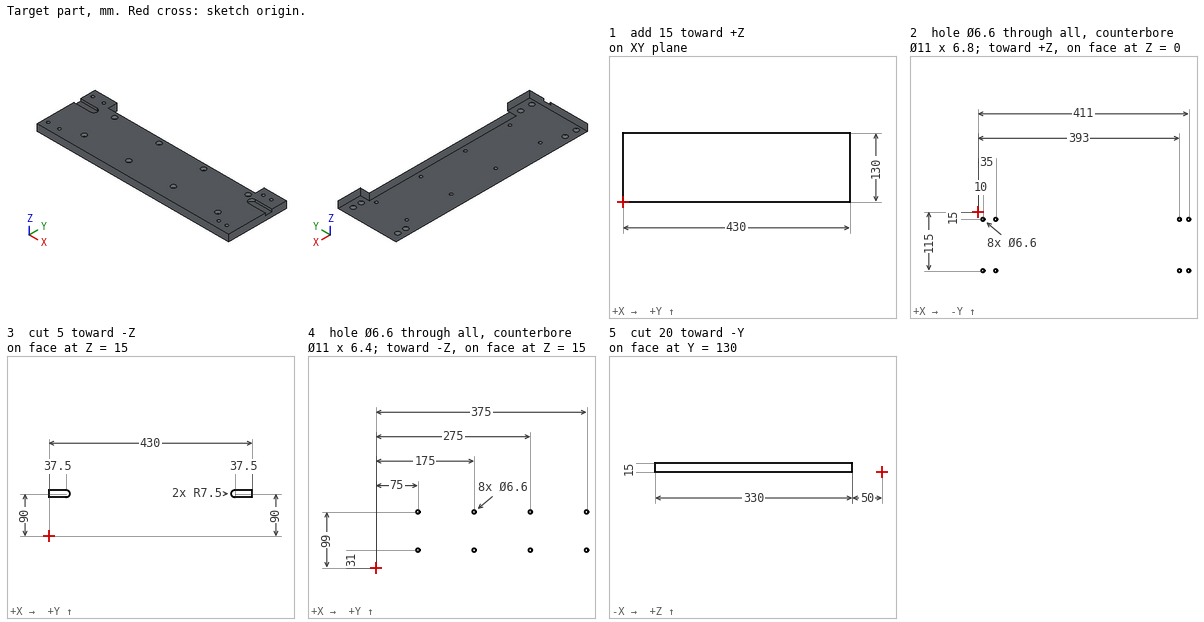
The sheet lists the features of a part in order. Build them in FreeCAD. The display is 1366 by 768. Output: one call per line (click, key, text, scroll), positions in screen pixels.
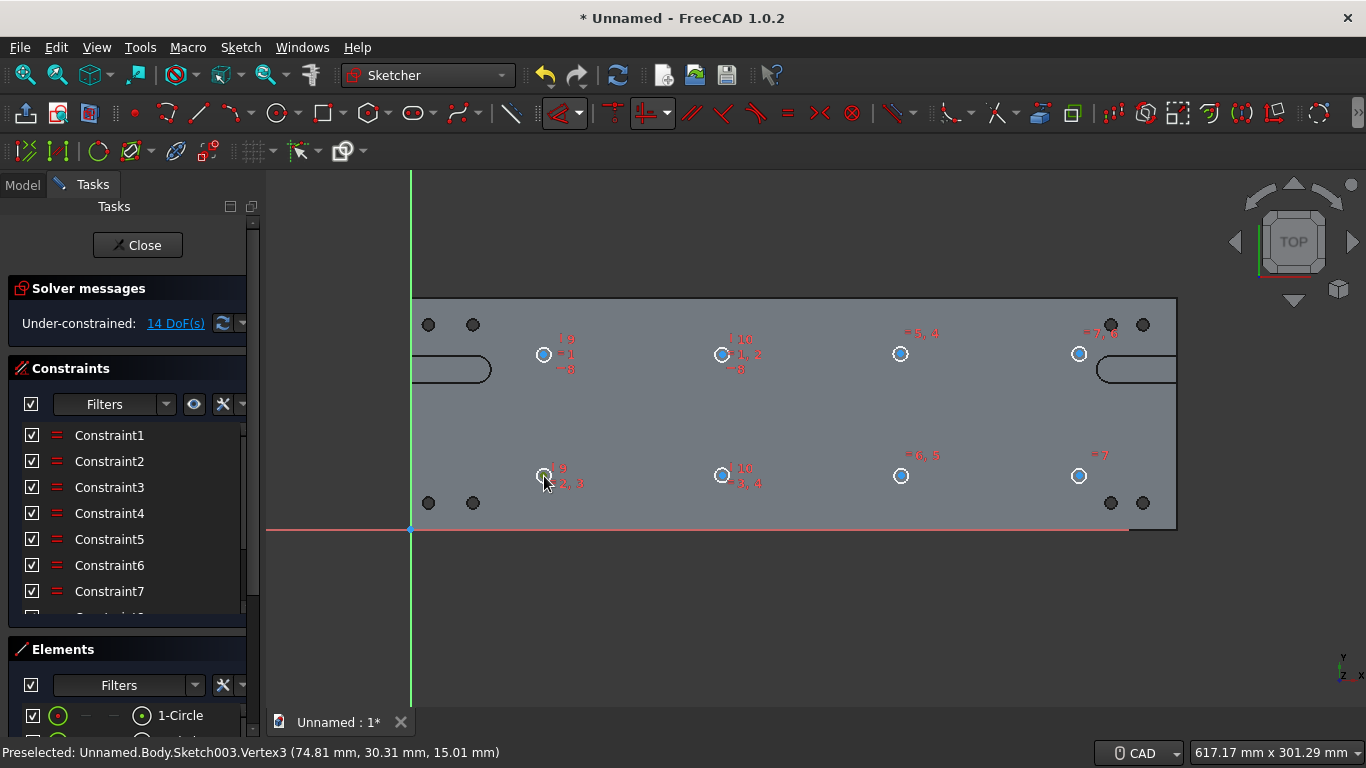
click(722, 475)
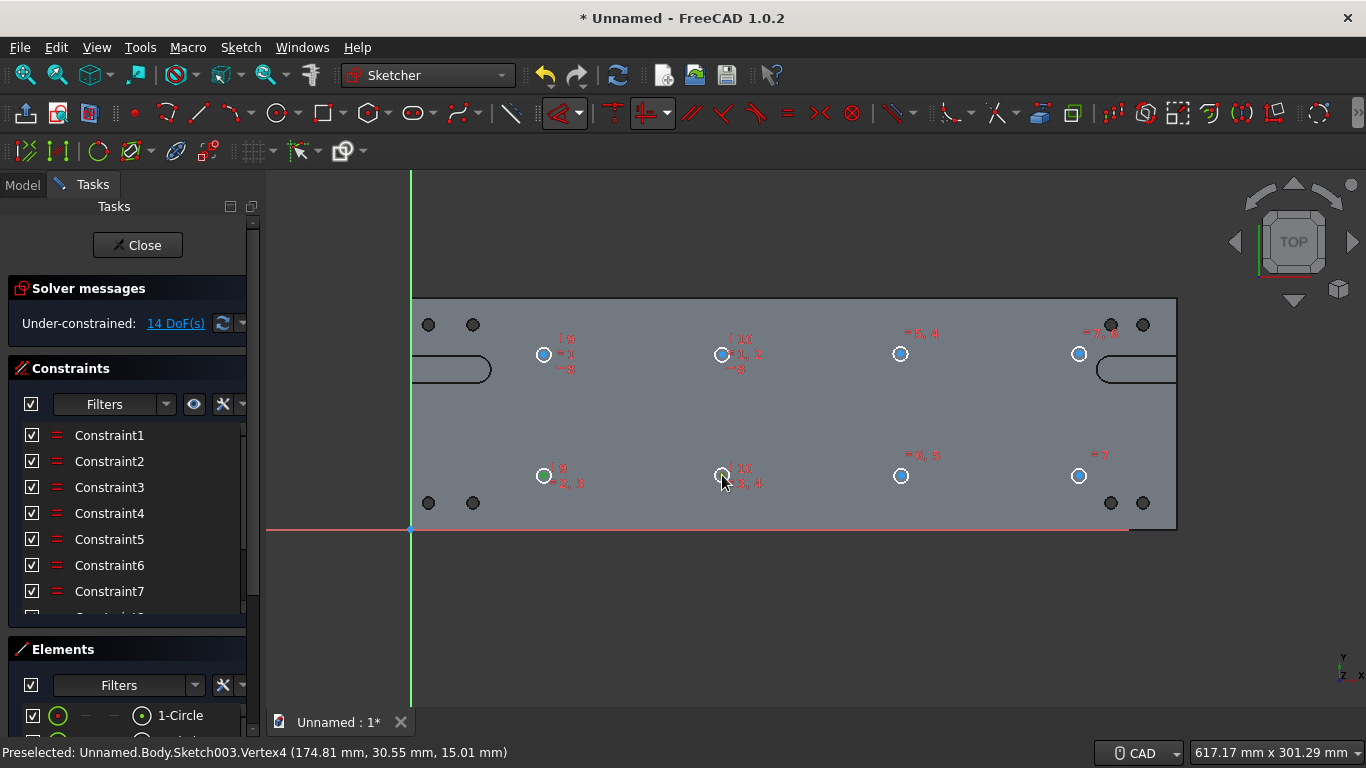
key(h)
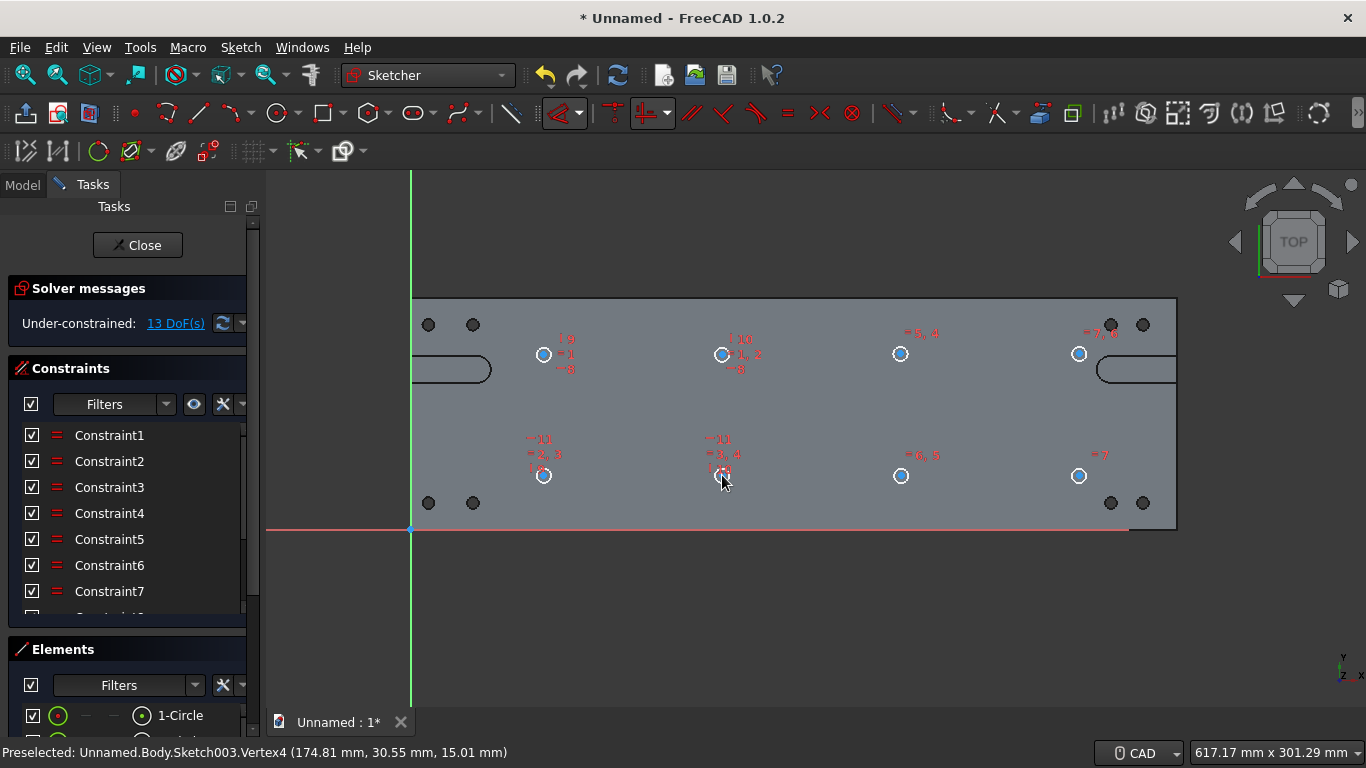
click(722, 355)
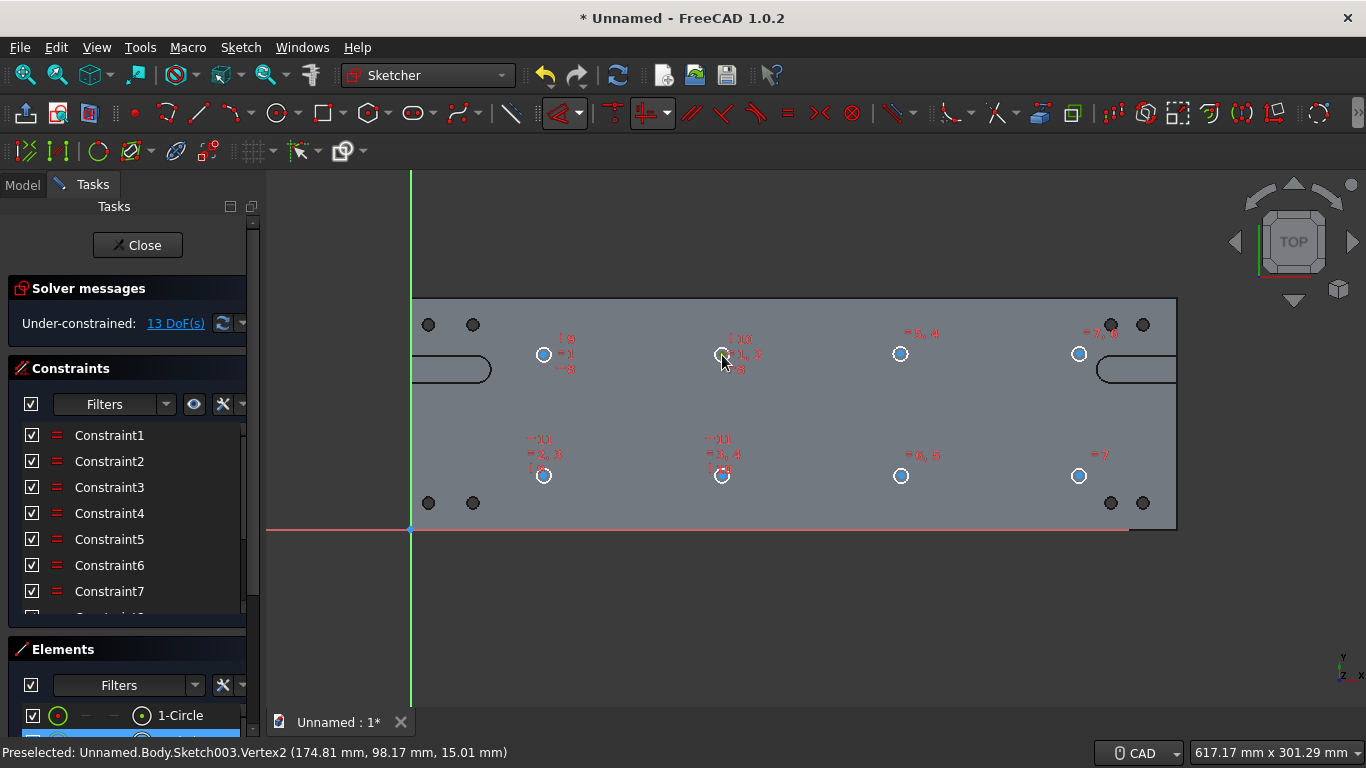
click(900, 354)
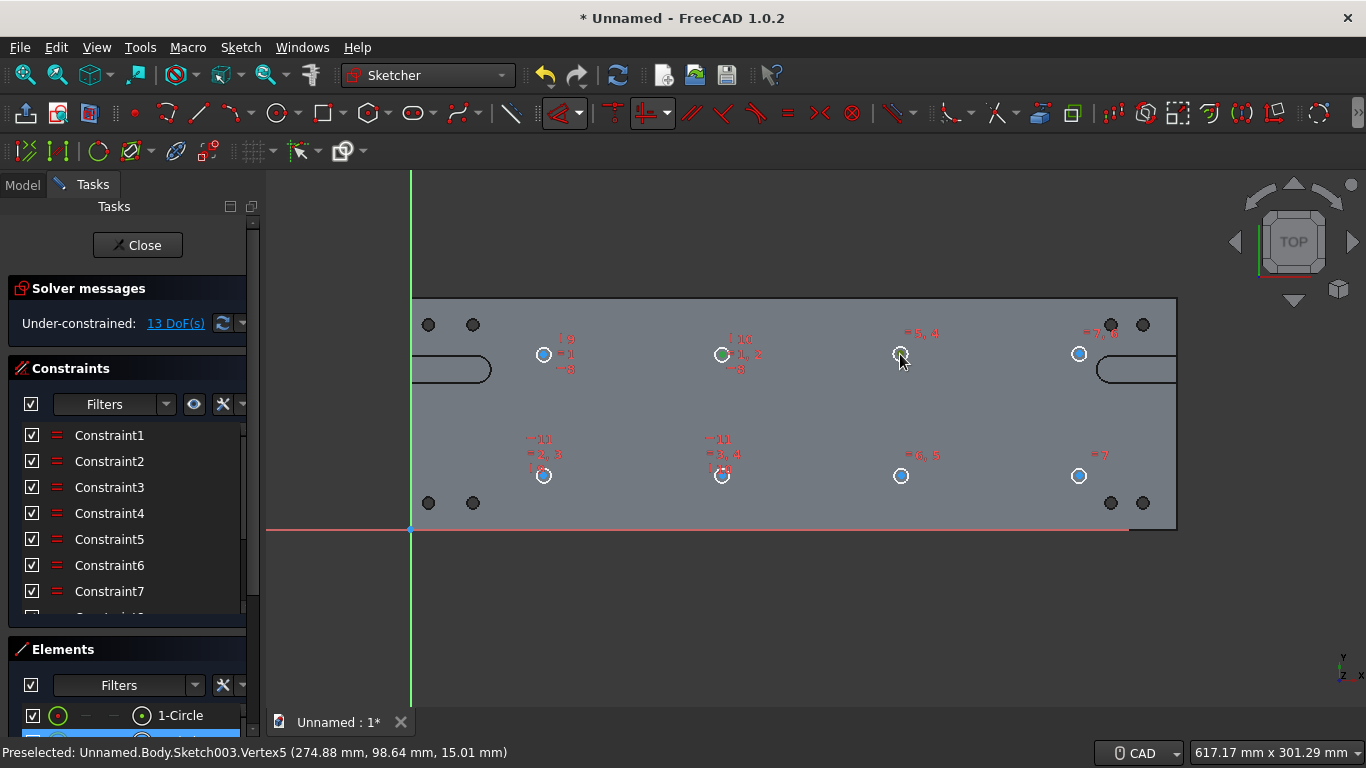
key(h)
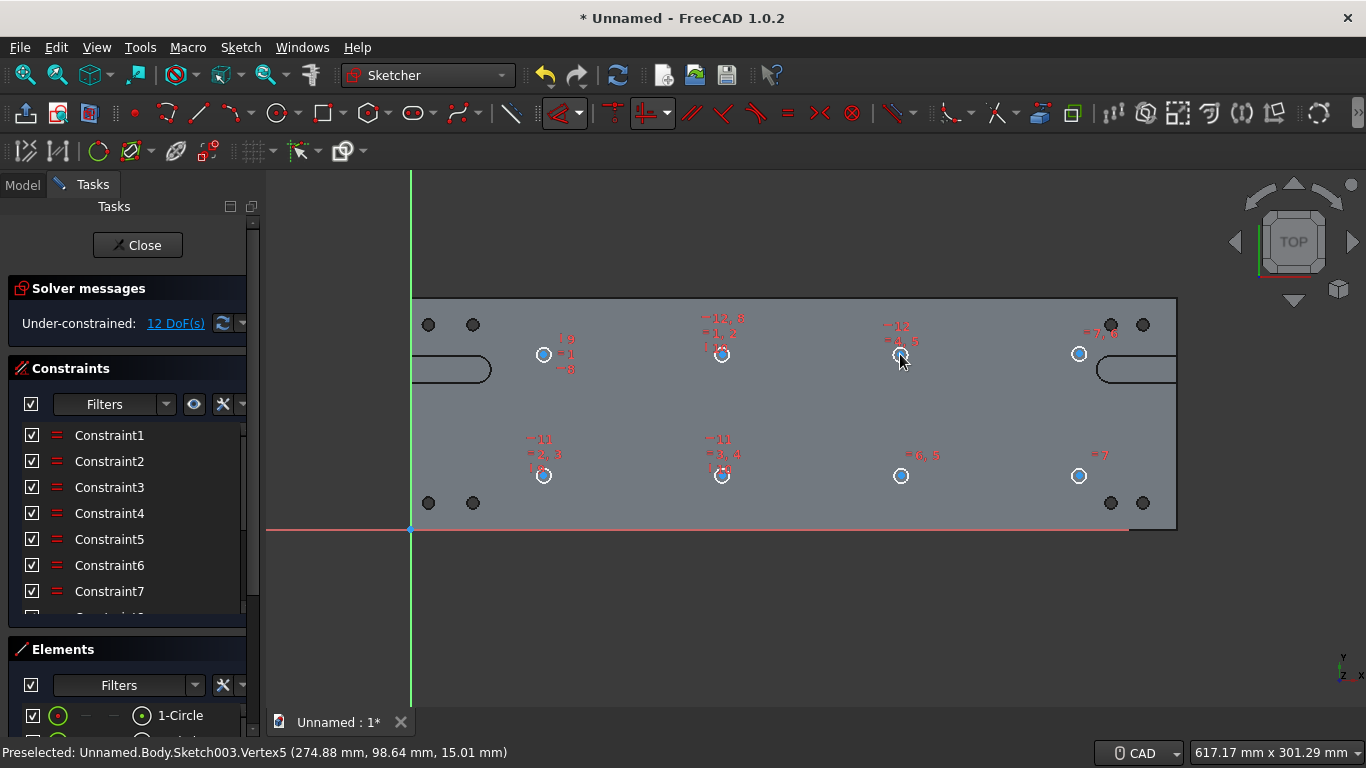
click(900, 355)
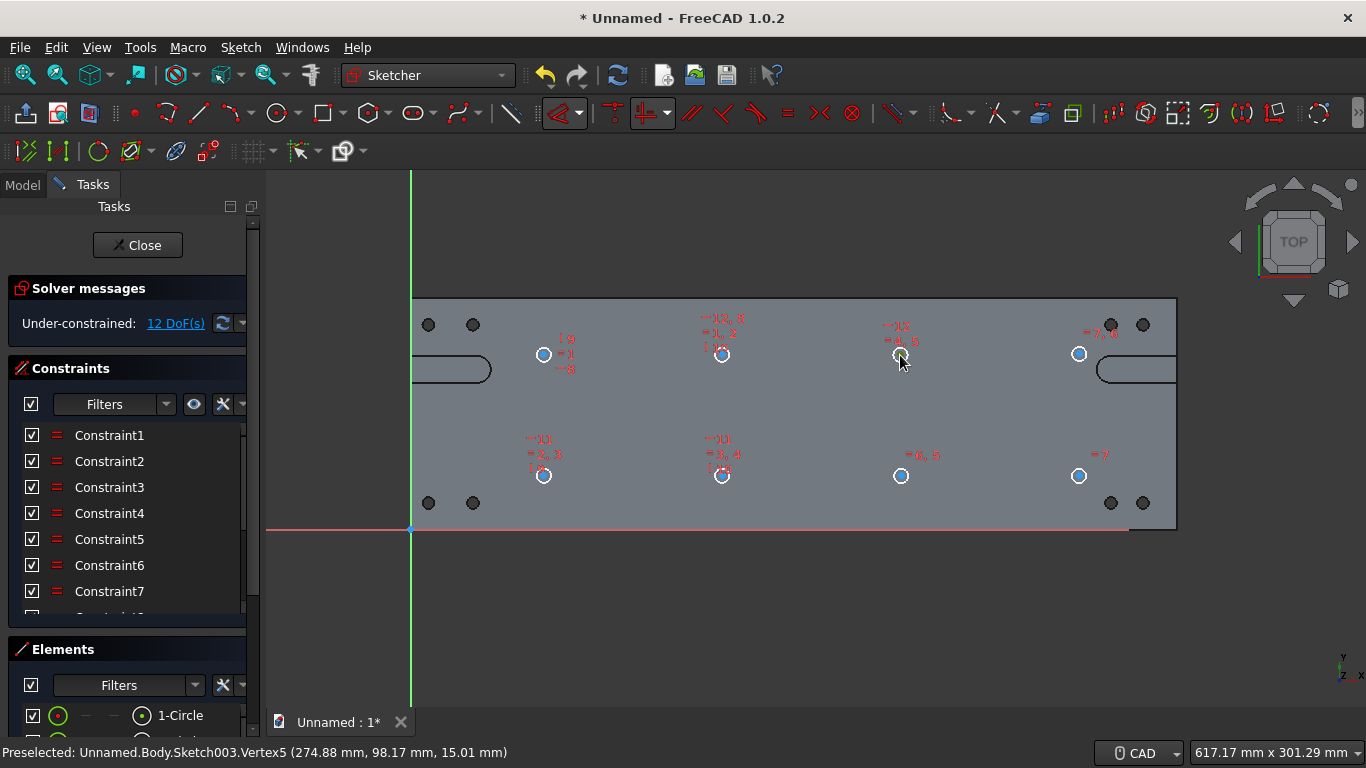
click(901, 476)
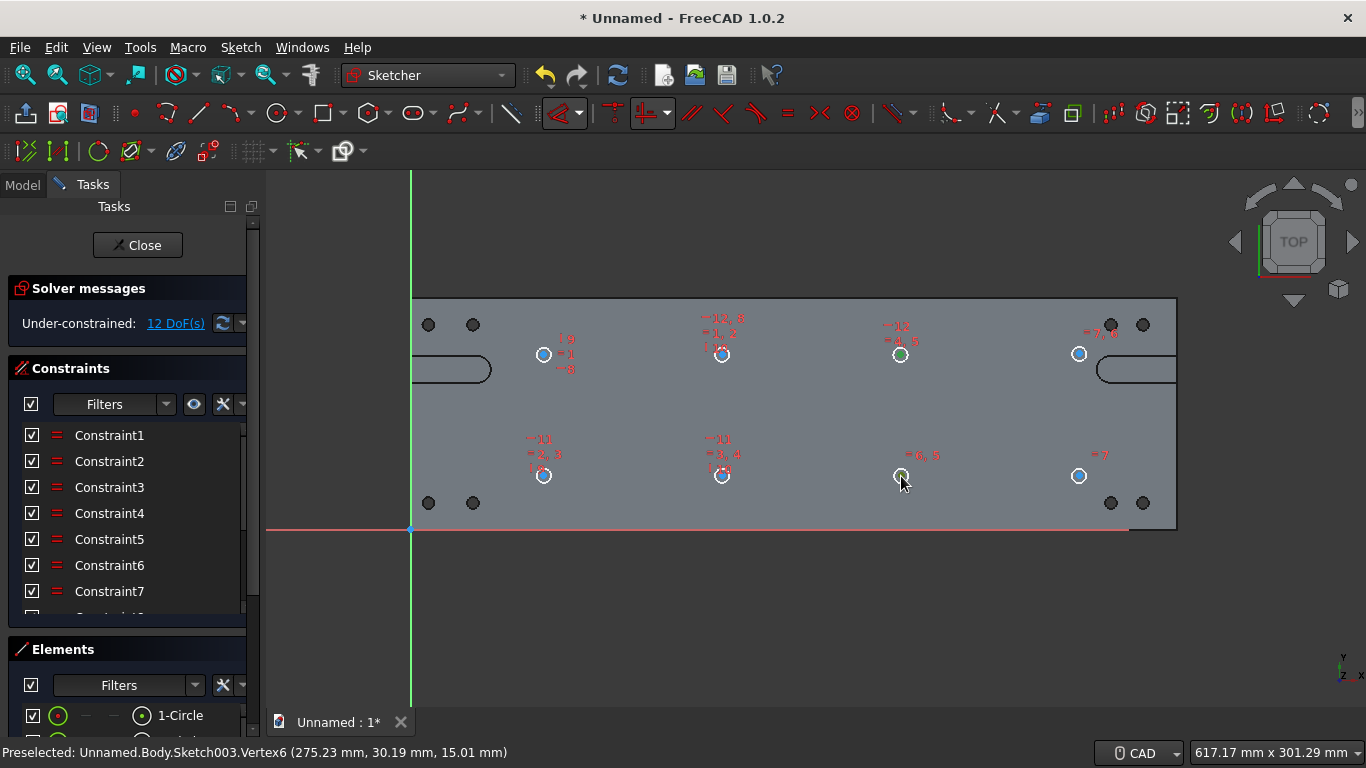
click(670, 114)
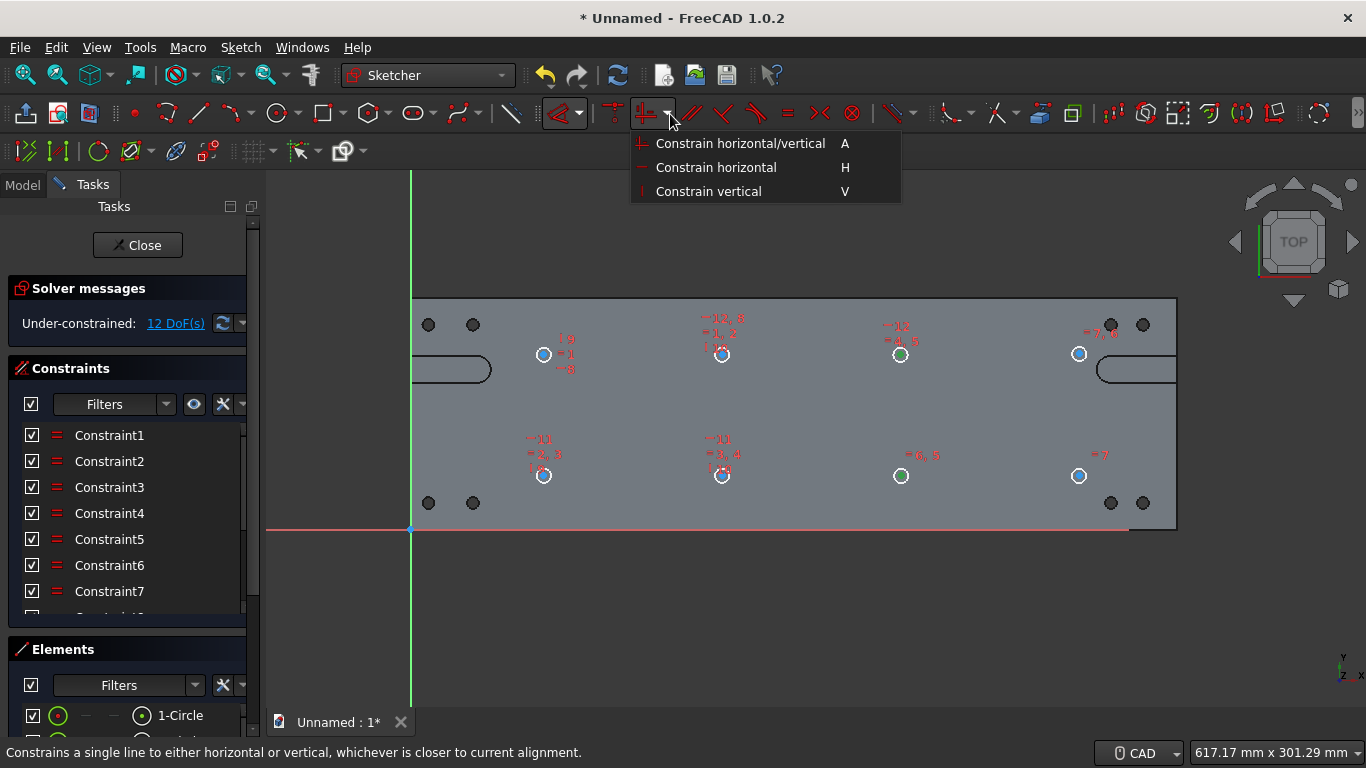
click(766, 191)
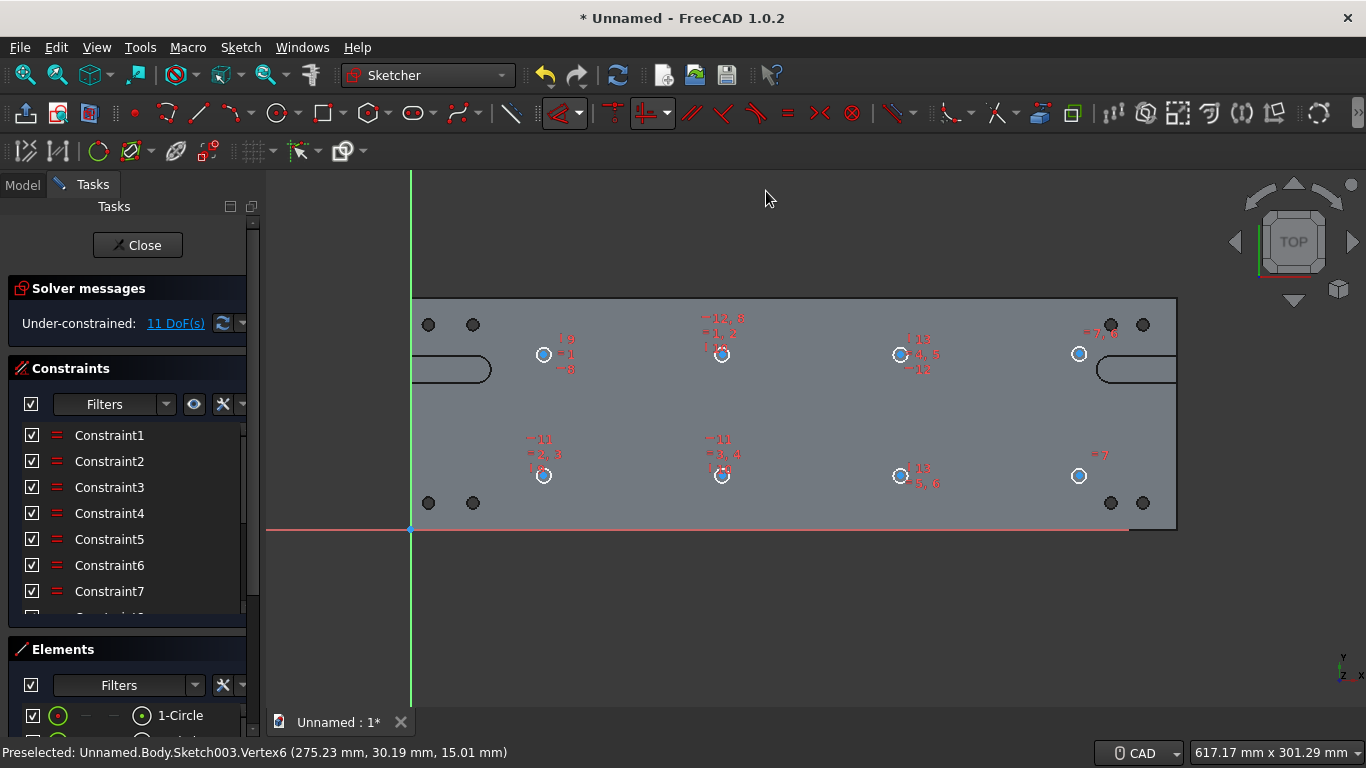
click(722, 476)